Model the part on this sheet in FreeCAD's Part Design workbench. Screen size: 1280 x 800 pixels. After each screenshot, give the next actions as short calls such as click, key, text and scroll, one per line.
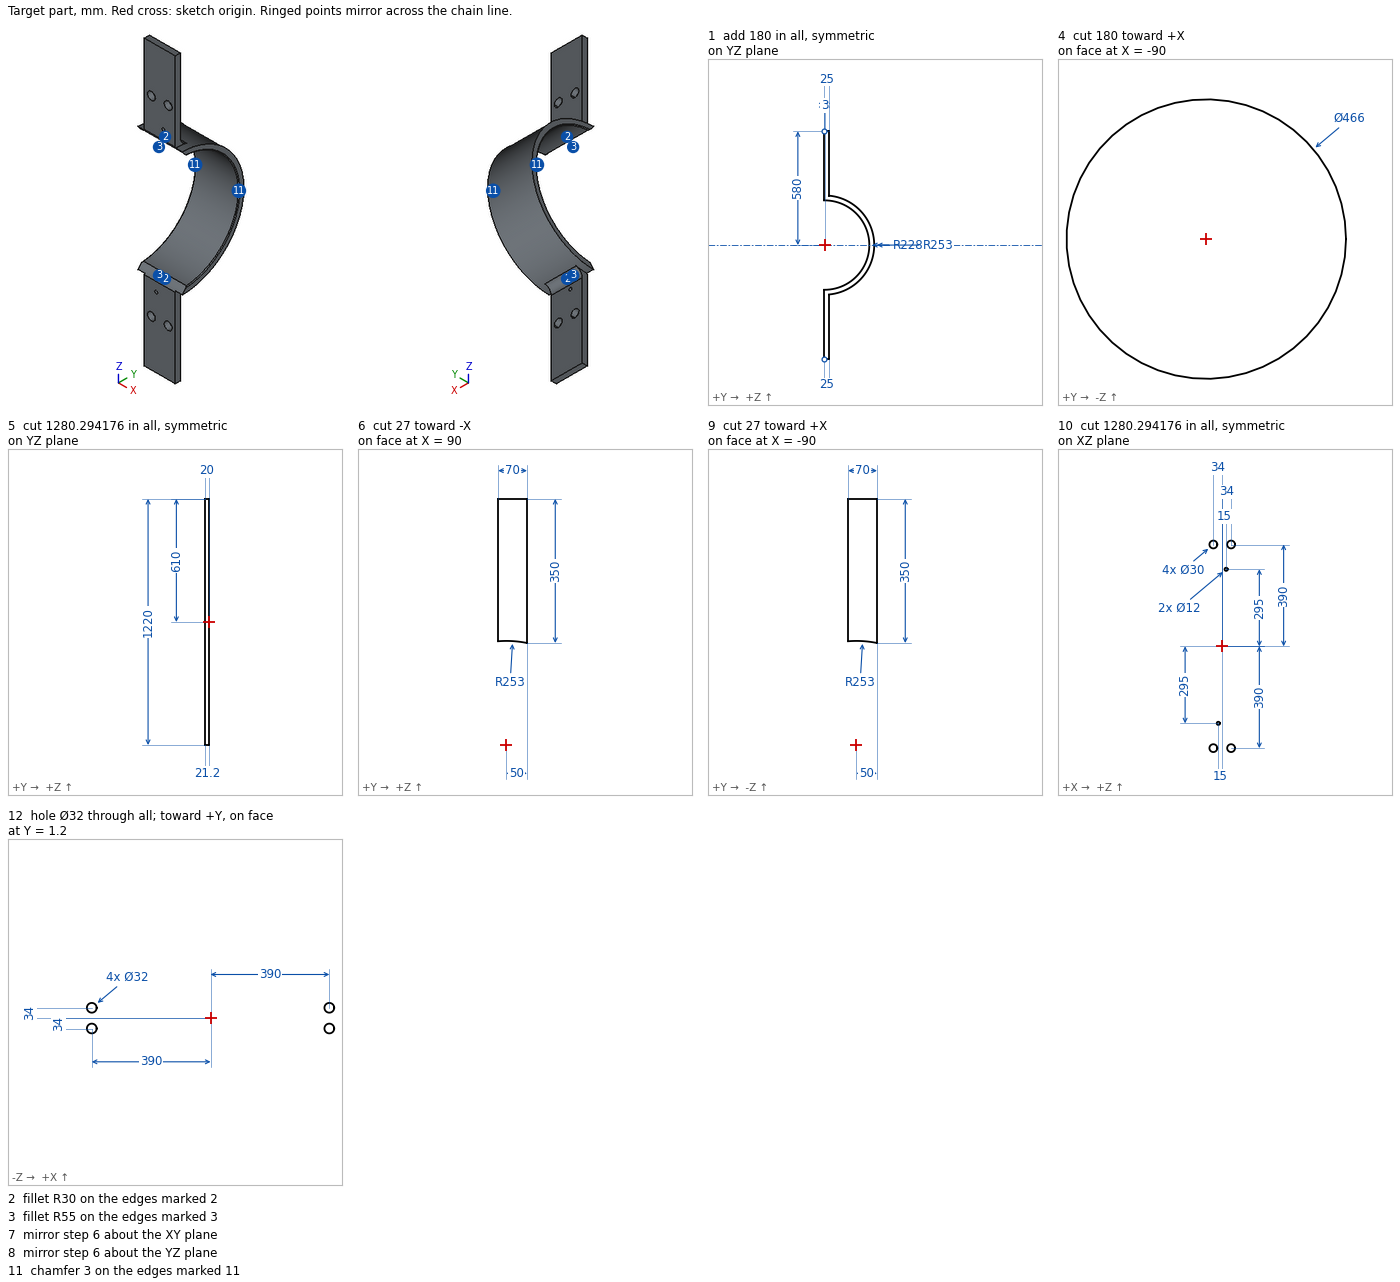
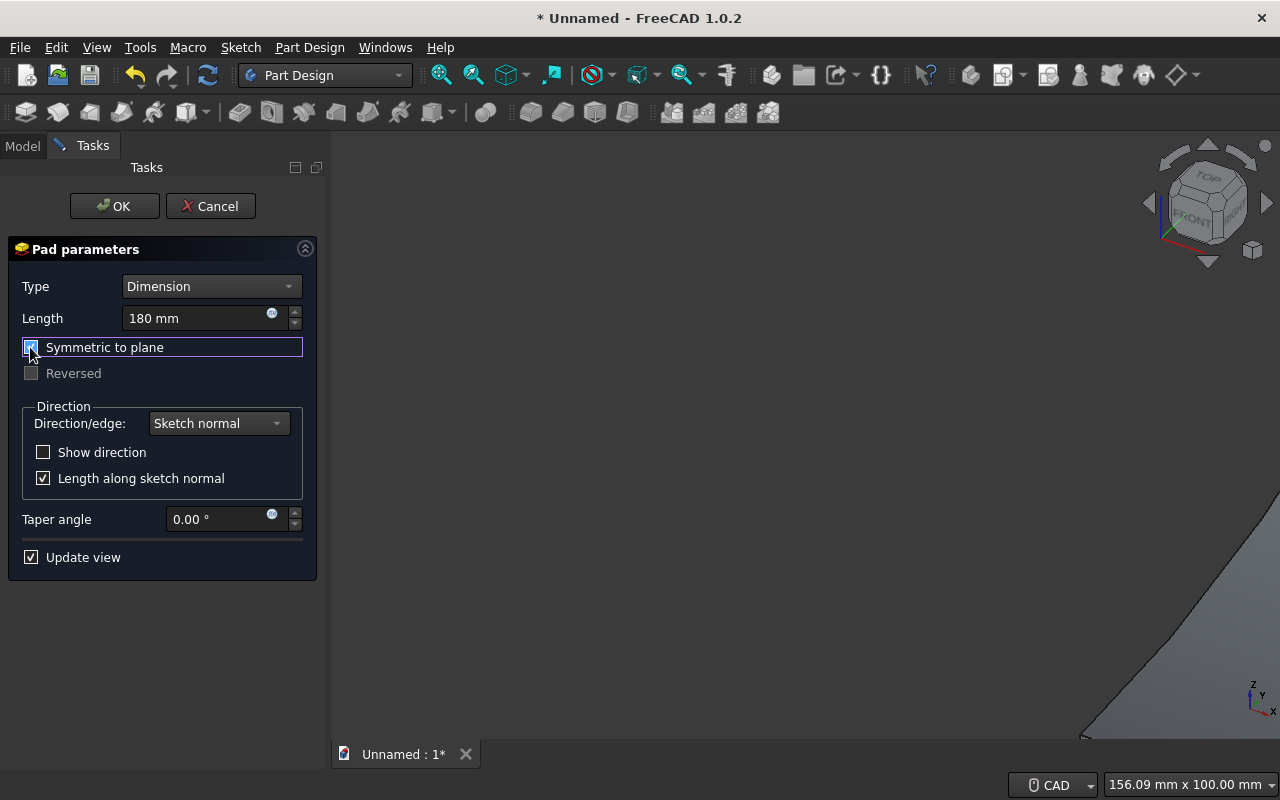
click(115, 206)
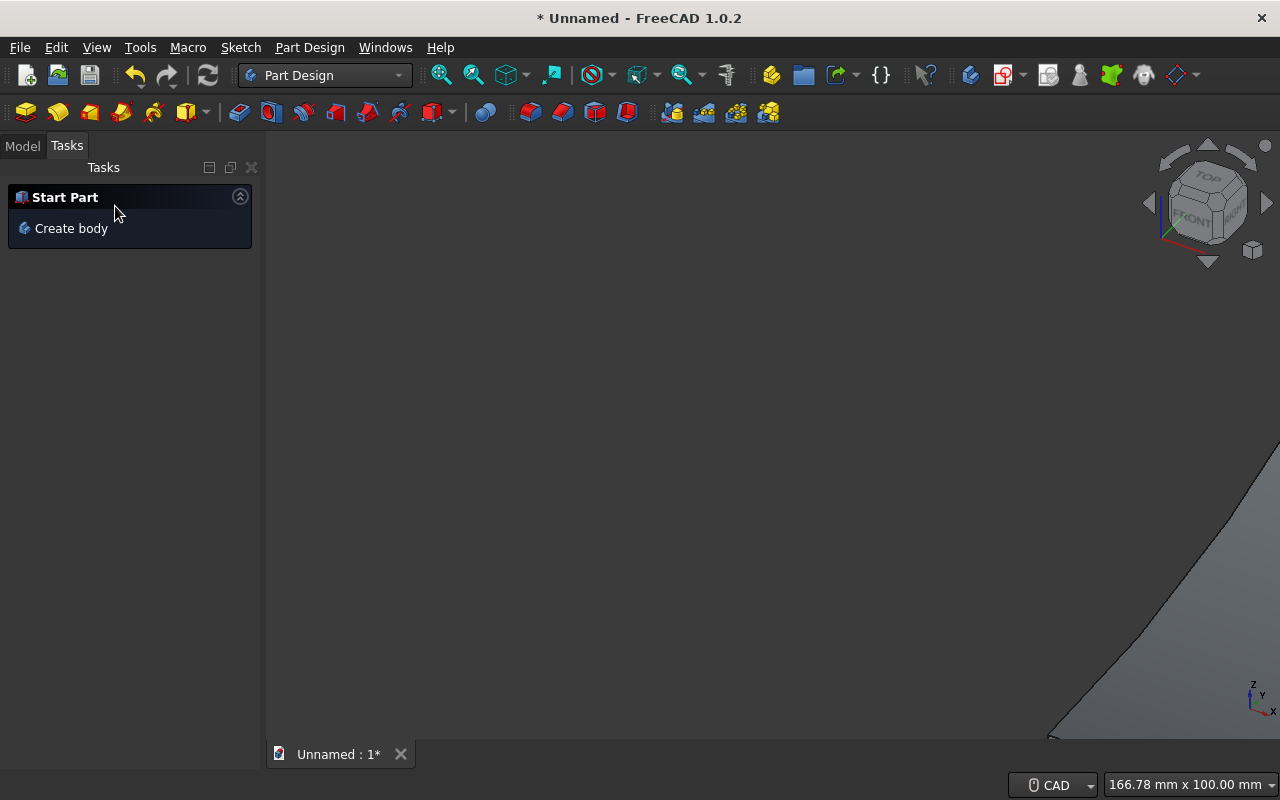
click(442, 76)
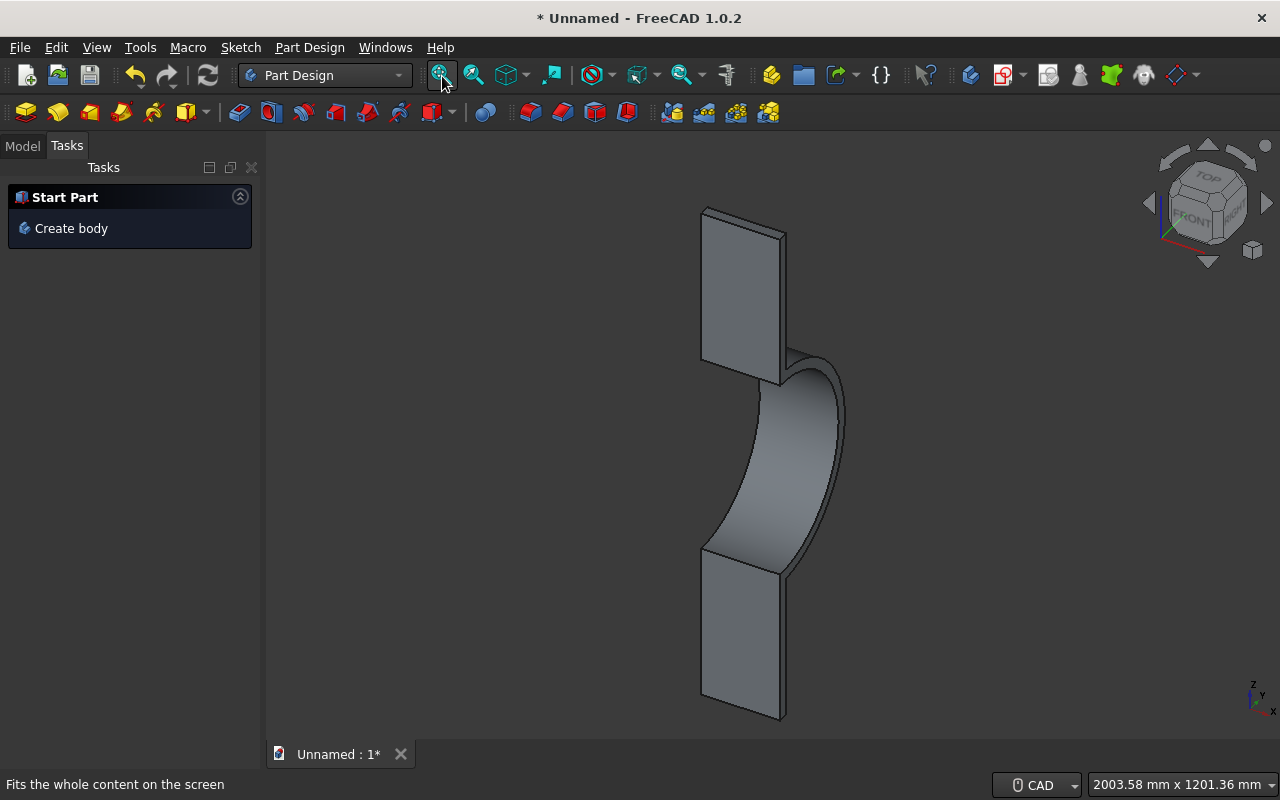
key(0)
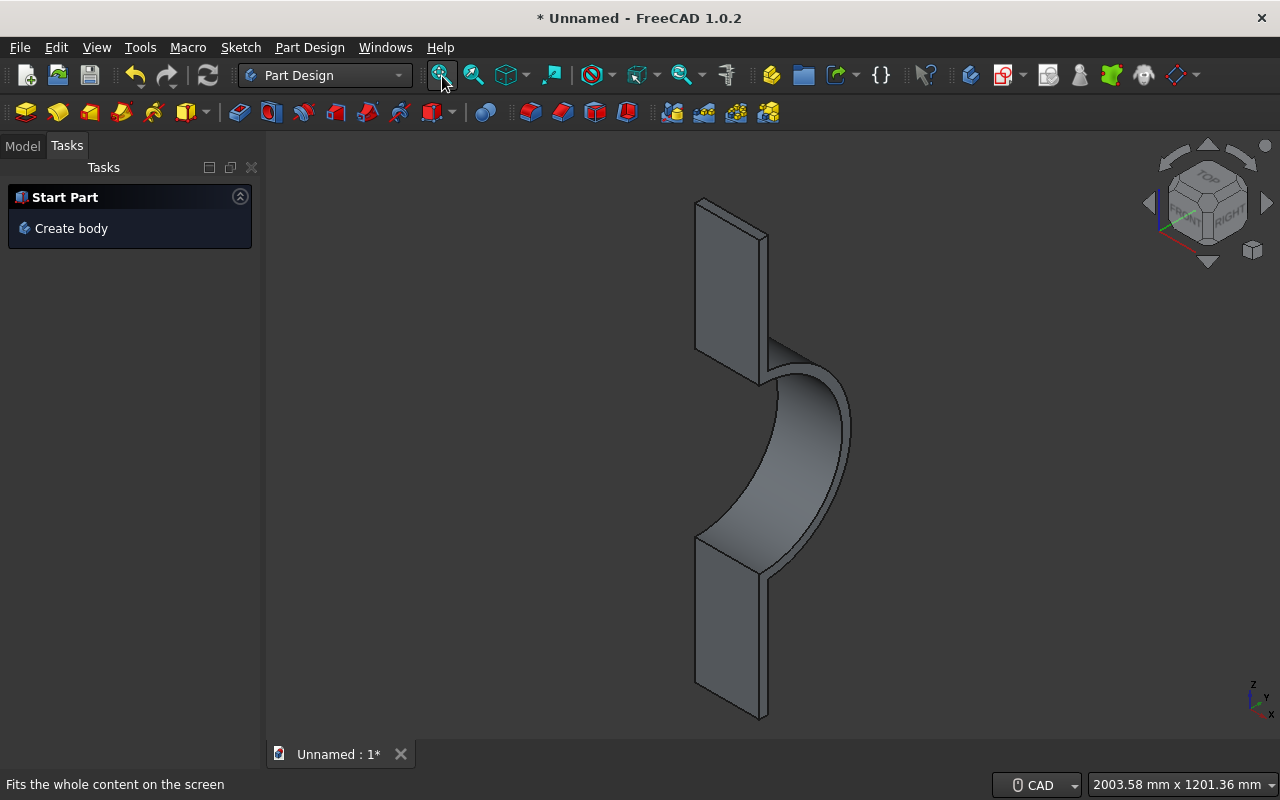
key(2)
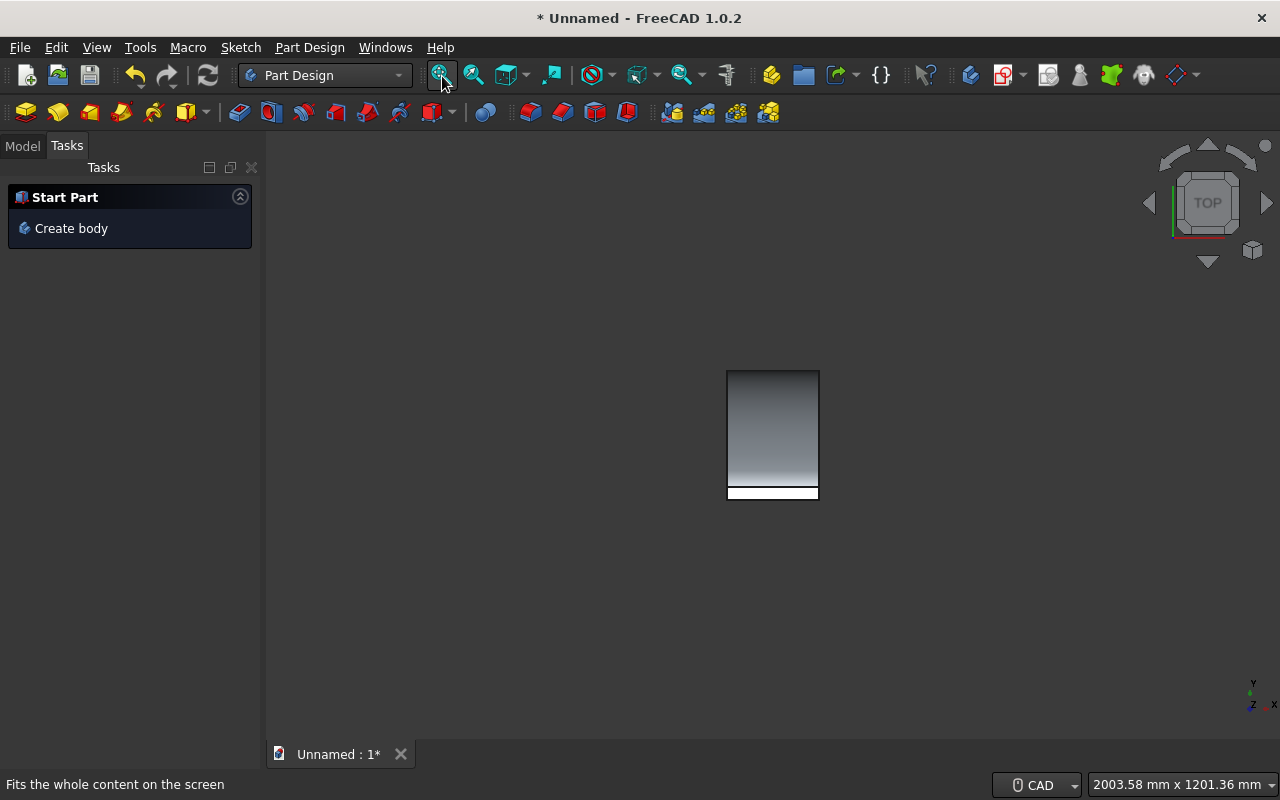
click(442, 76)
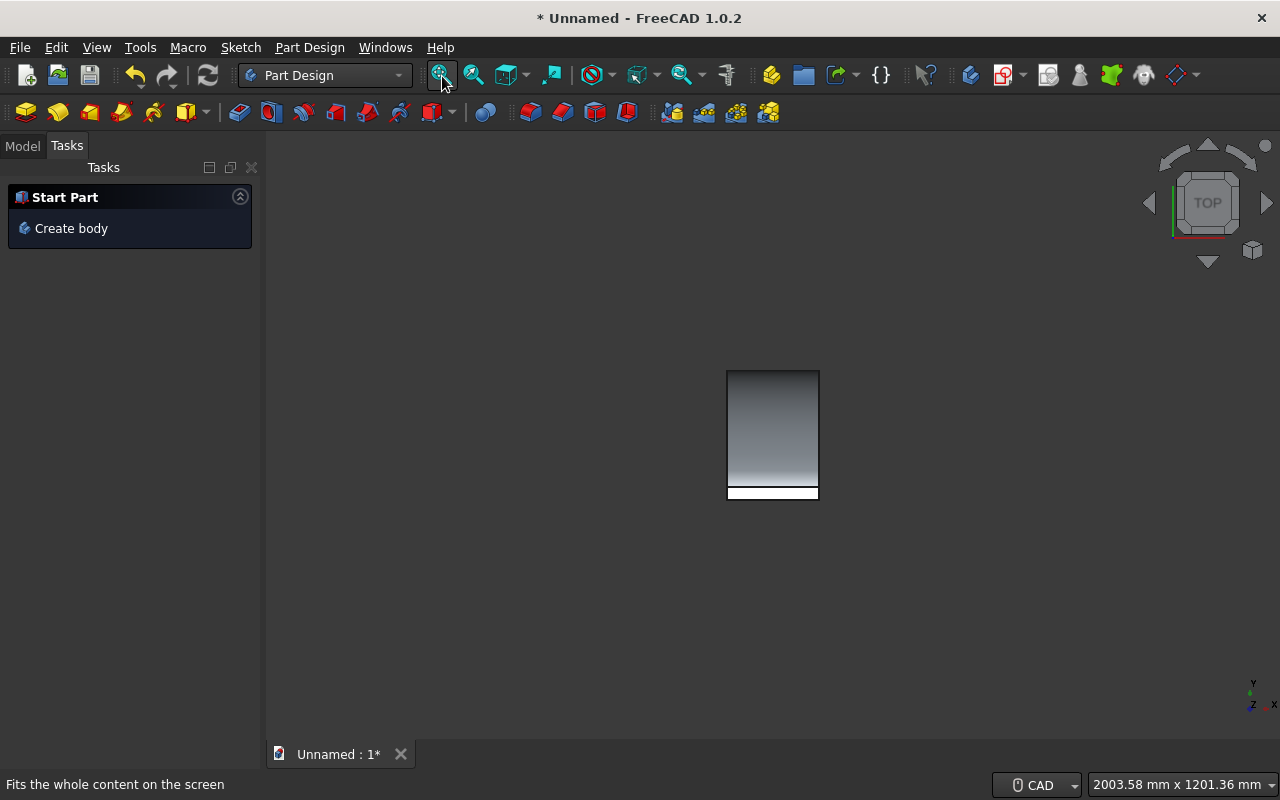
key(1)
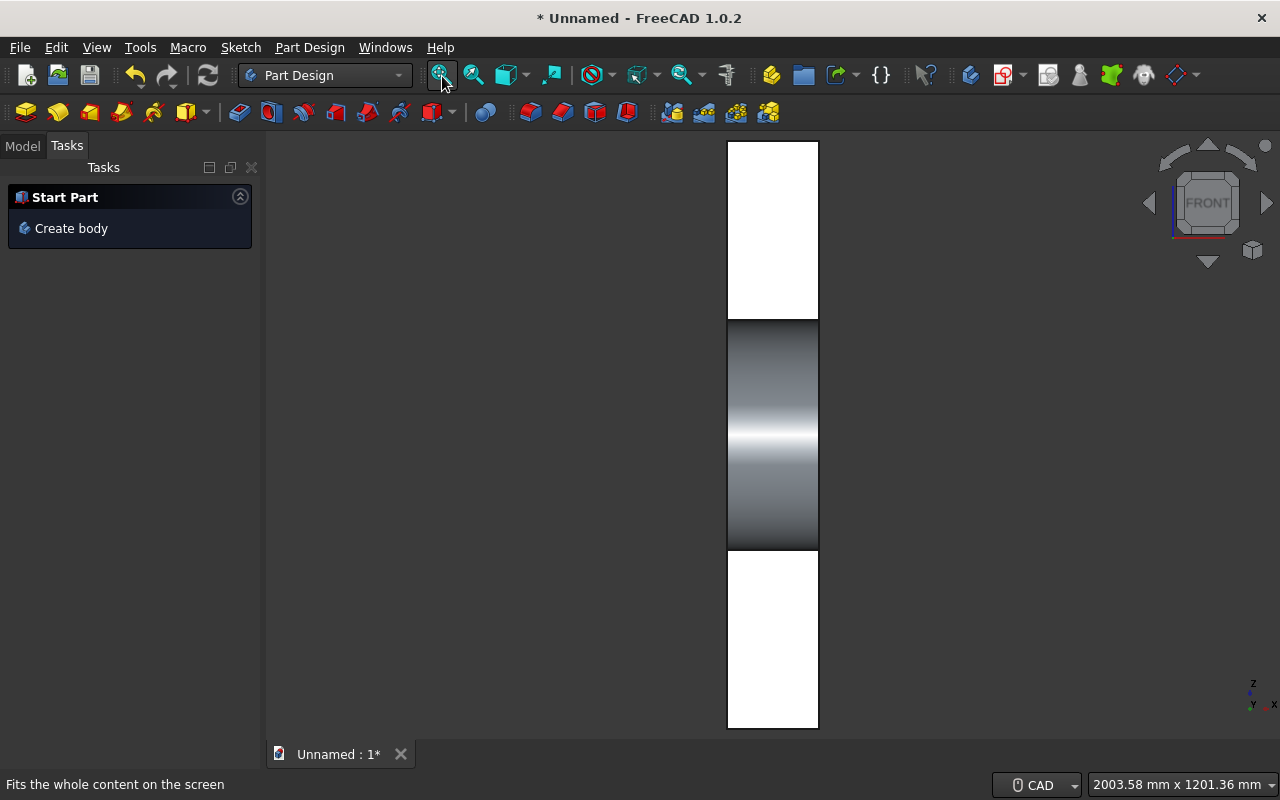
key(3)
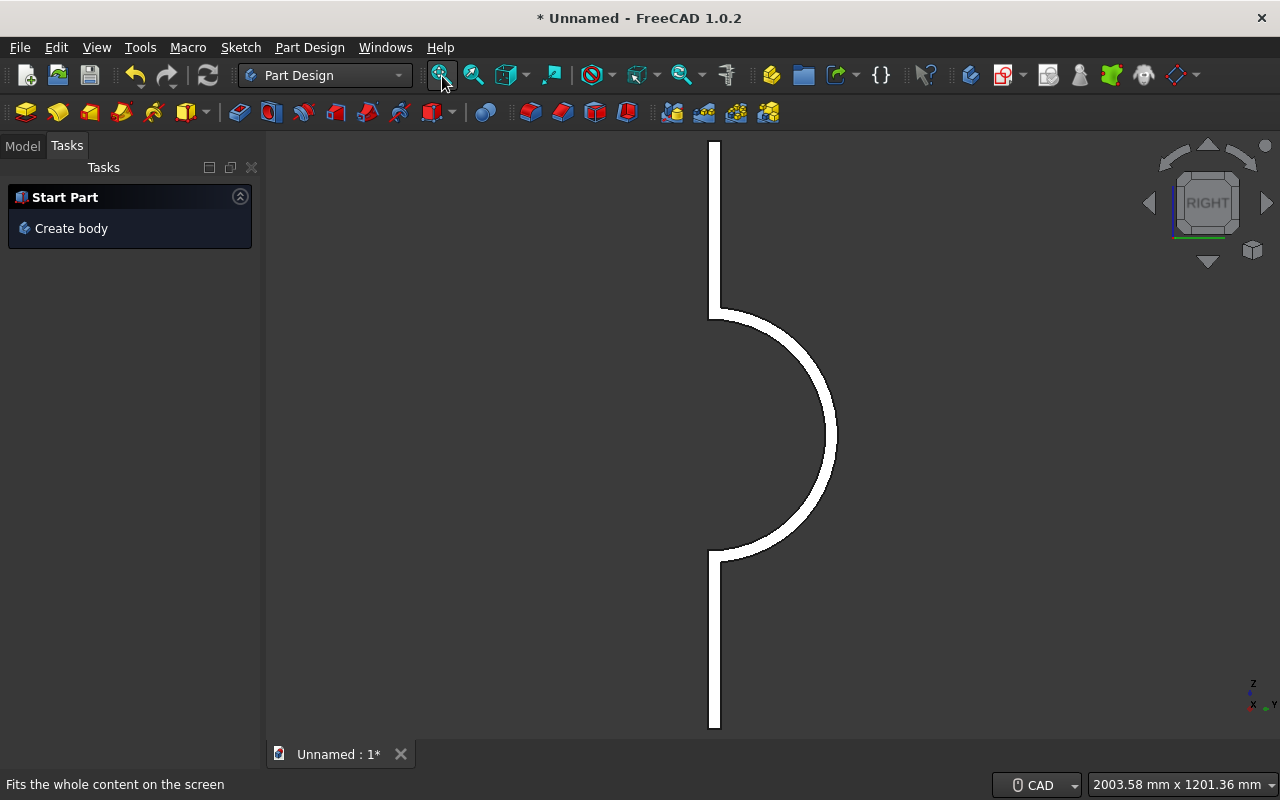
key(5)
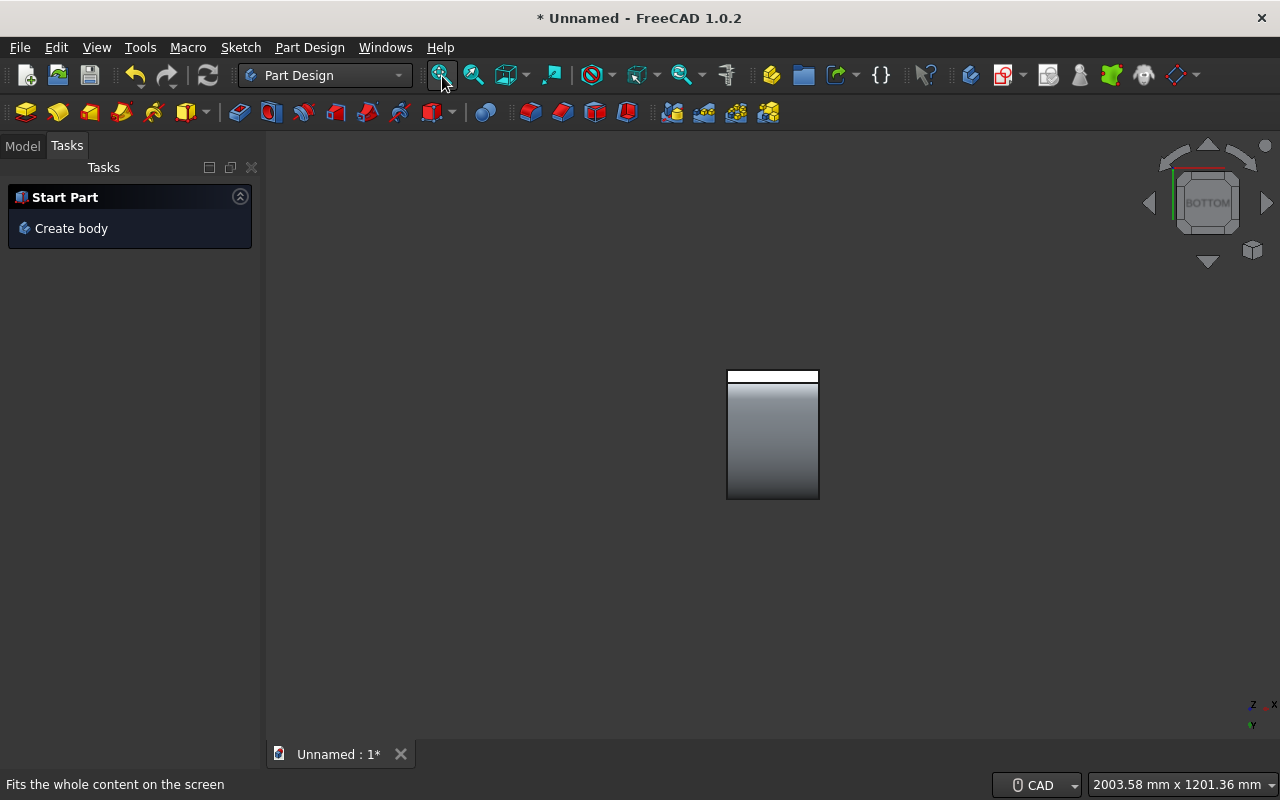
click(442, 76)